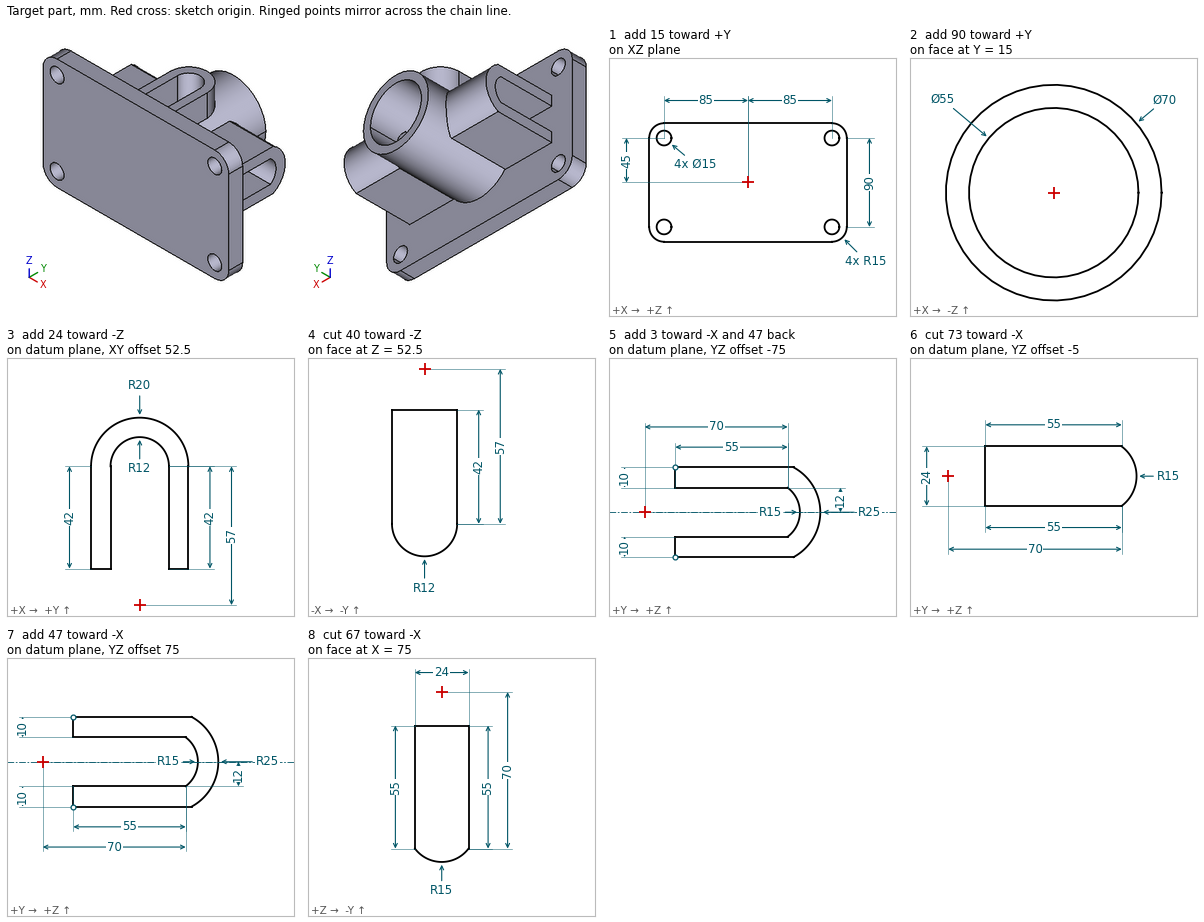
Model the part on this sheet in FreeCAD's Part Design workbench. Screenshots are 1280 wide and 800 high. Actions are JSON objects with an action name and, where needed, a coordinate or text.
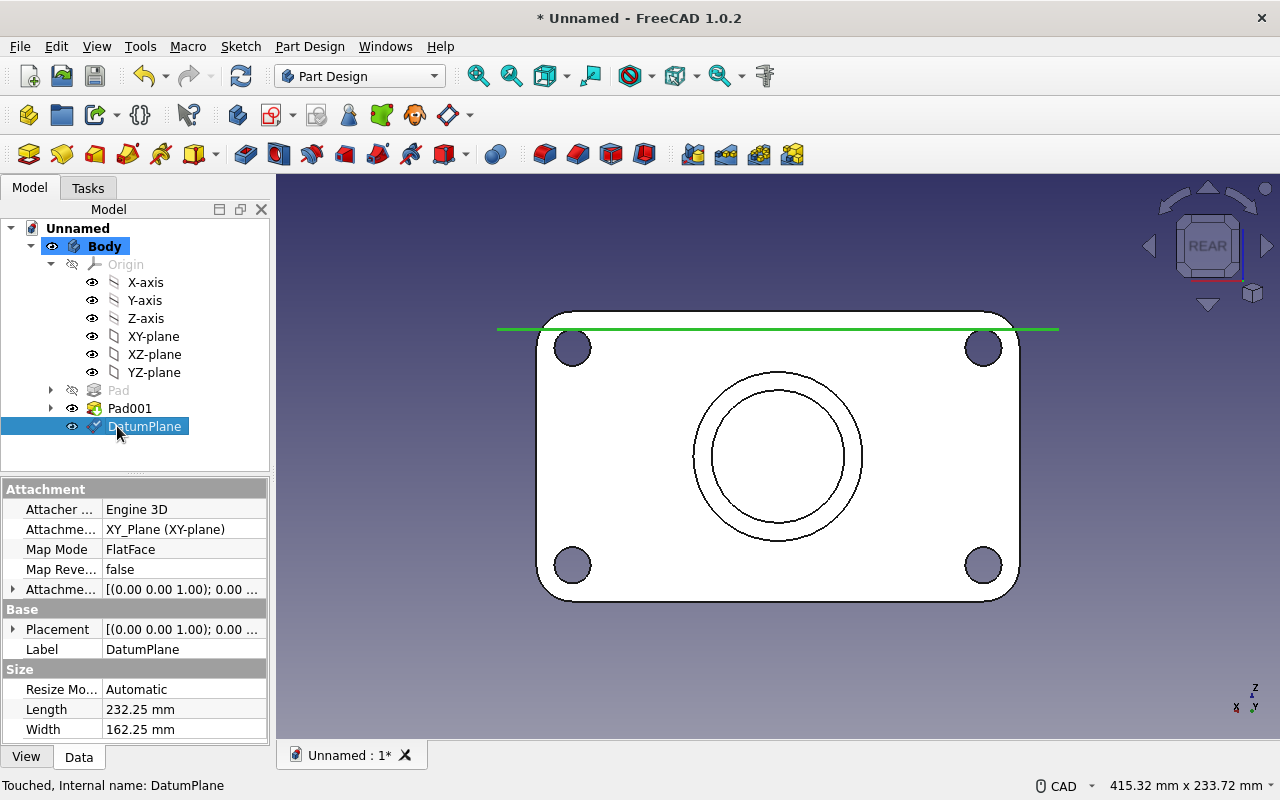
{"action": "left_click", "coordinate": [270, 116]}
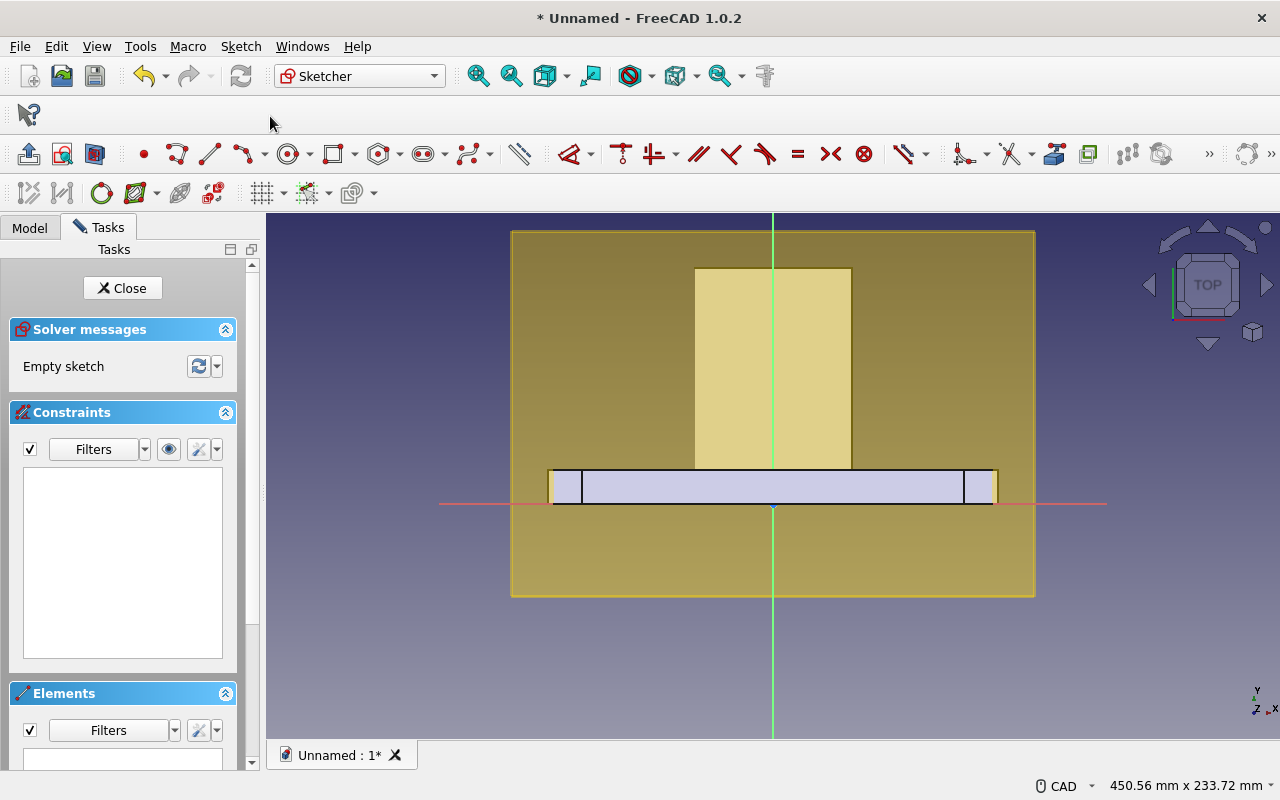
{"action": "key", "text": "q s"}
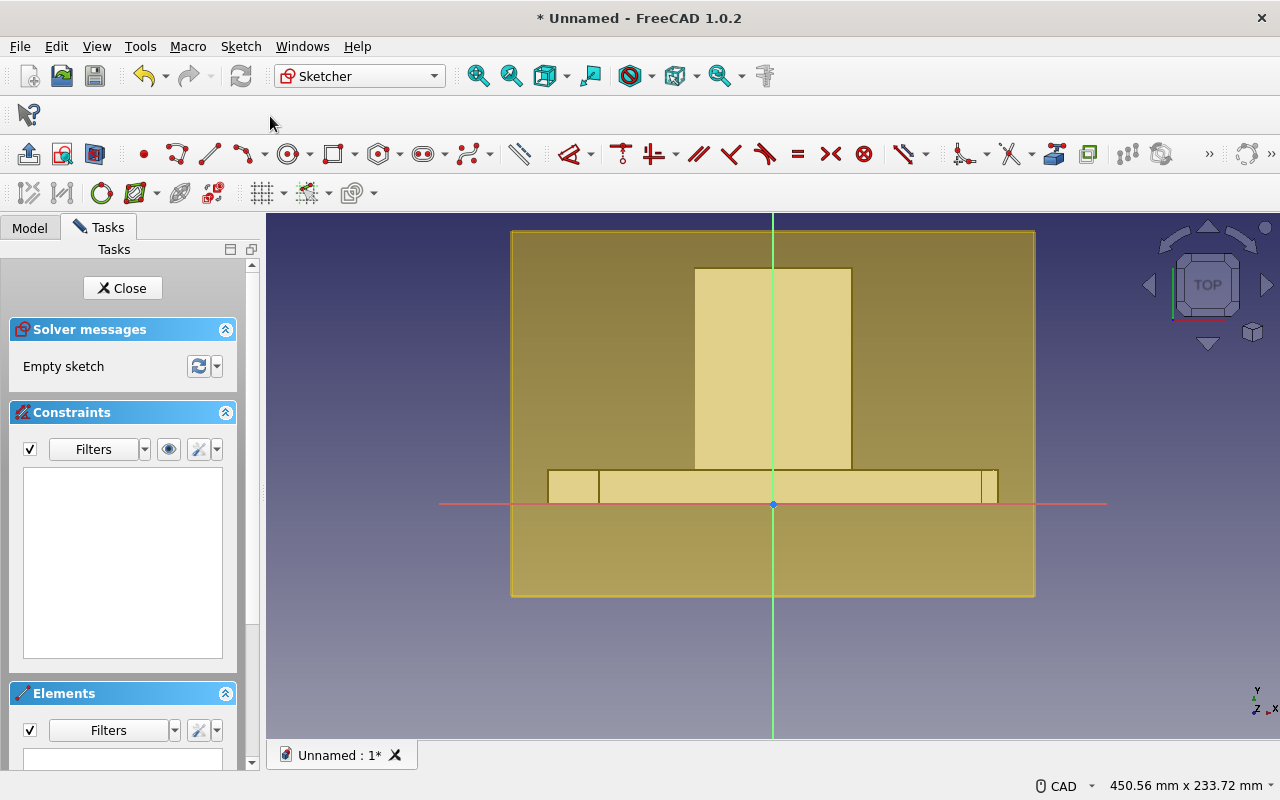
{"action": "scroll", "coordinate": [856, 346], "scroll_direction": "up", "scroll_amount": 3}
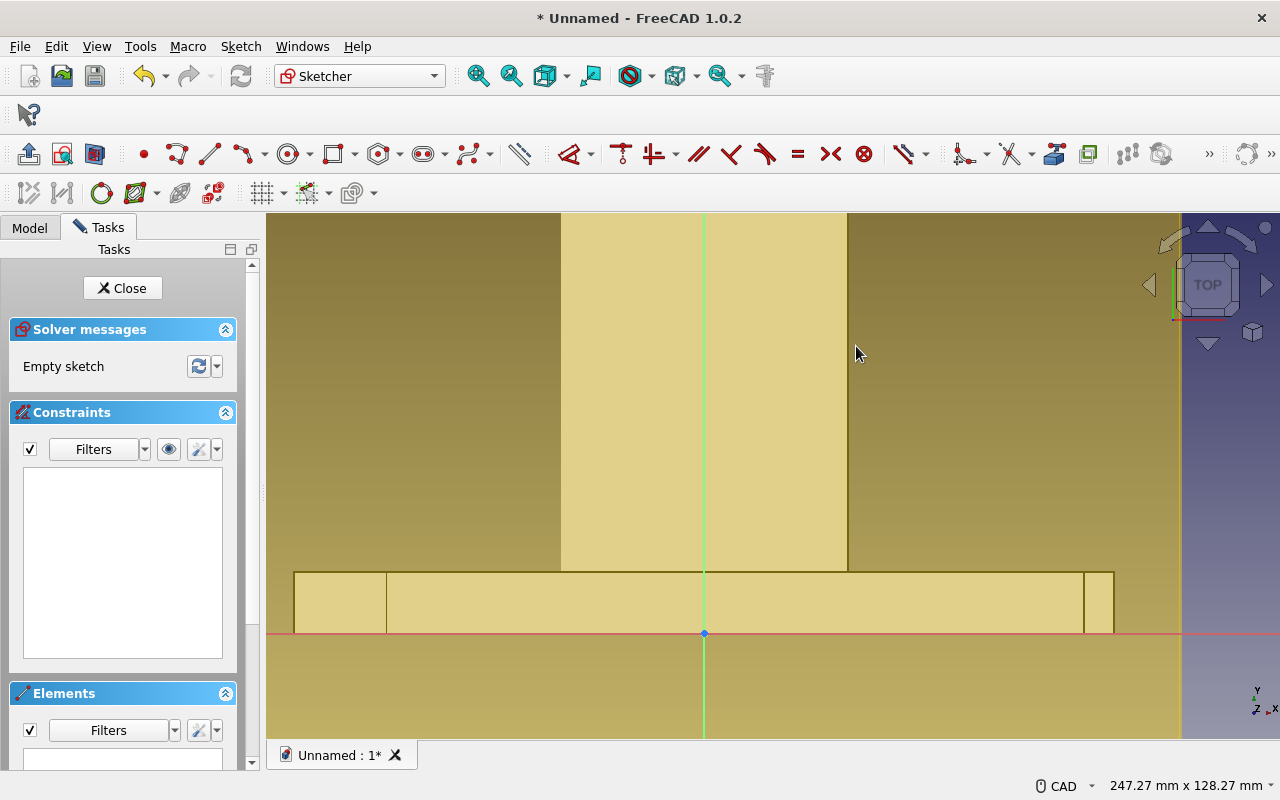
{"action": "key", "text": "g m"}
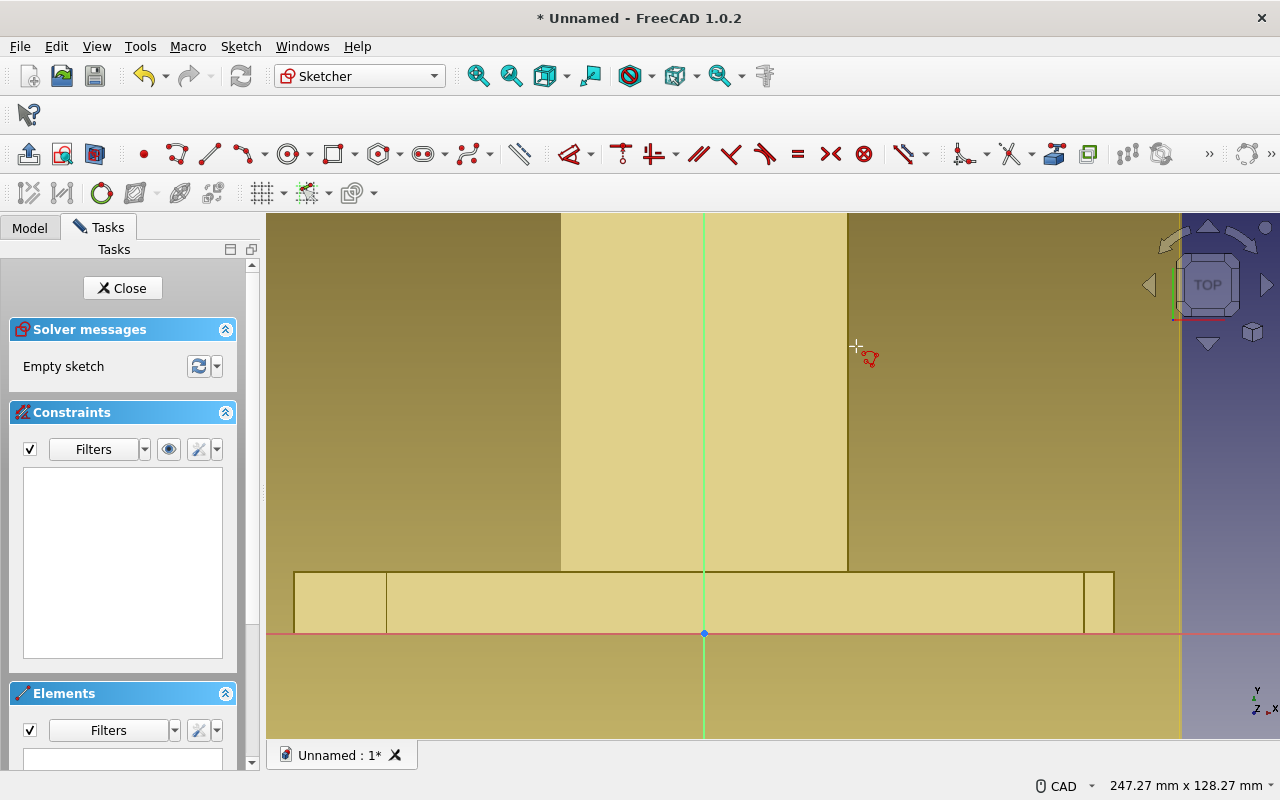
{"action": "left_click", "coordinate": [753, 400]}
{"action": "left_click", "coordinate": [753, 572]}
{"action": "left_click", "coordinate": [786, 572]}
{"action": "left_click", "coordinate": [786, 400]}
{"action": "right_click", "coordinate": [786, 400]}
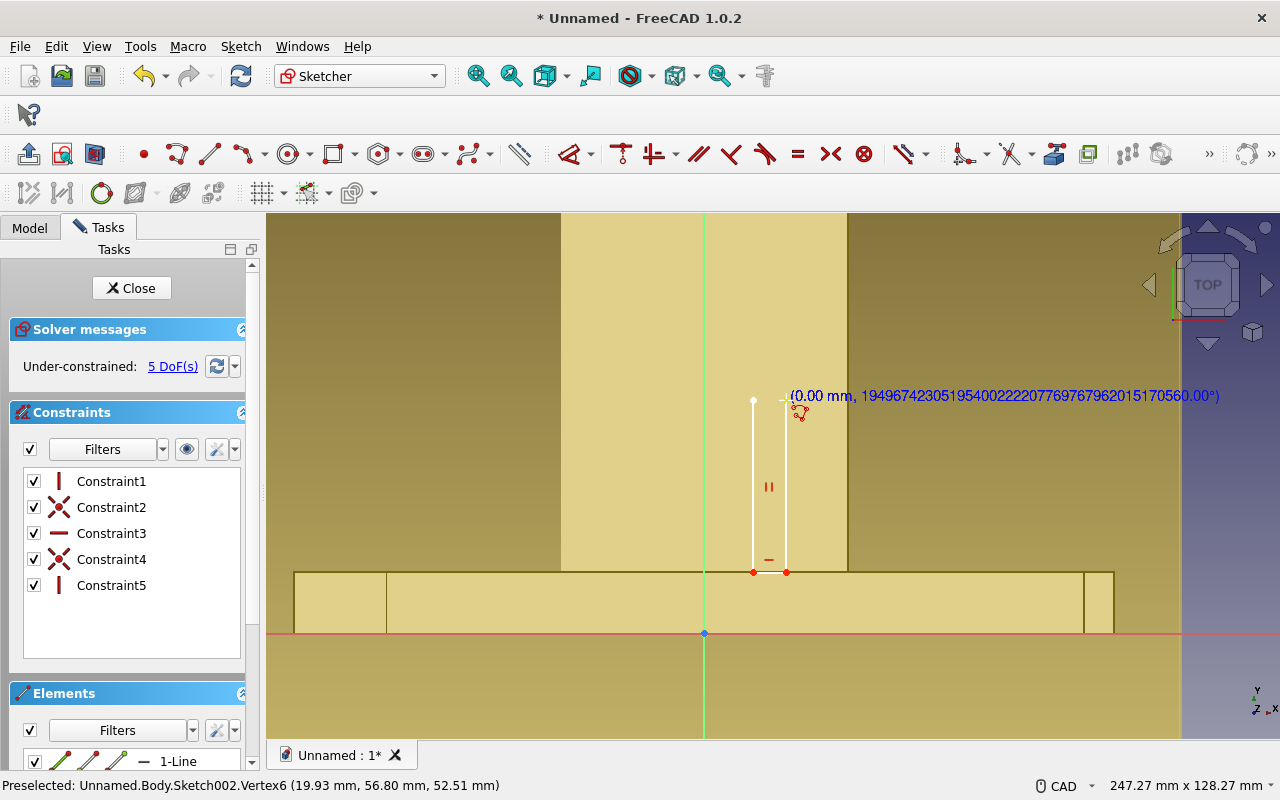
{"action": "left_click", "coordinate": [622, 400]}
{"action": "left_click", "coordinate": [622, 572]}
{"action": "left_click", "coordinate": [655, 572]}
{"action": "left_click", "coordinate": [655, 400]}
{"action": "right_click", "coordinate": [655, 400]}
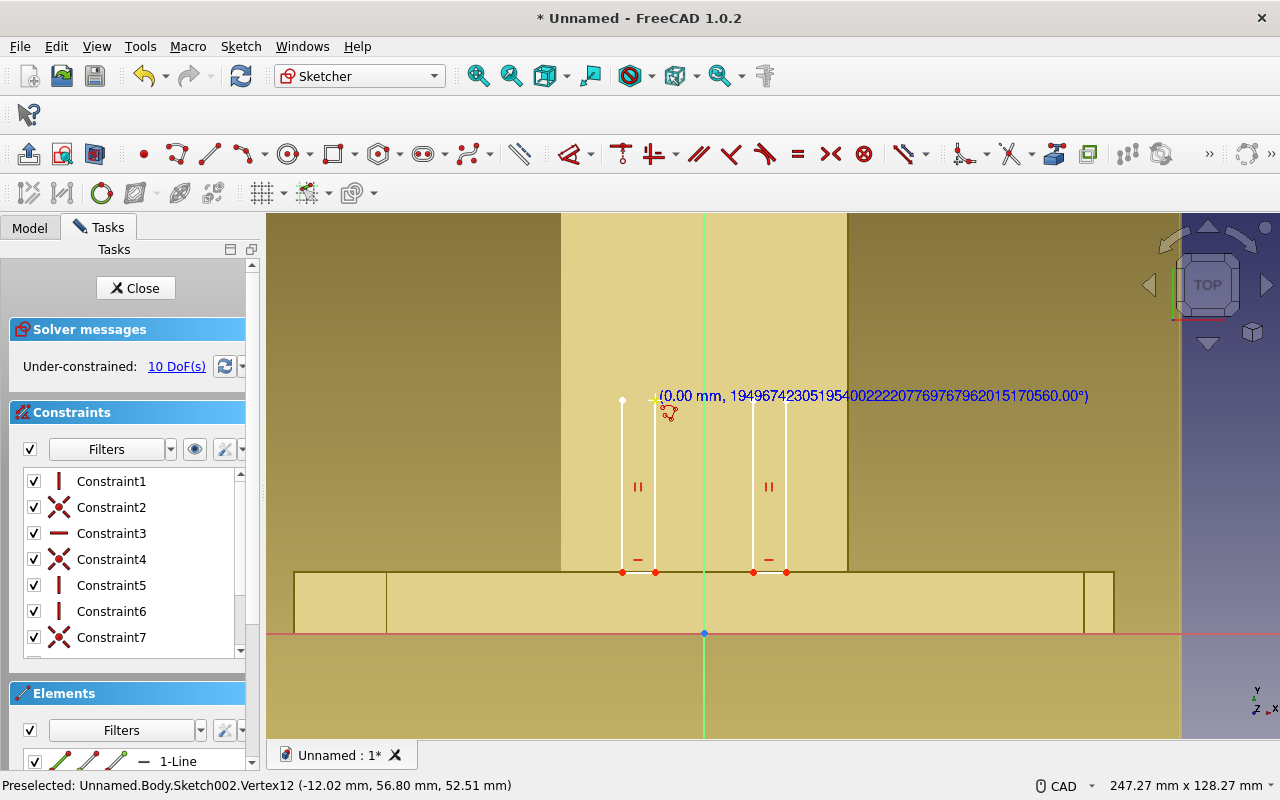
{"action": "left_click", "coordinate": [242, 154]}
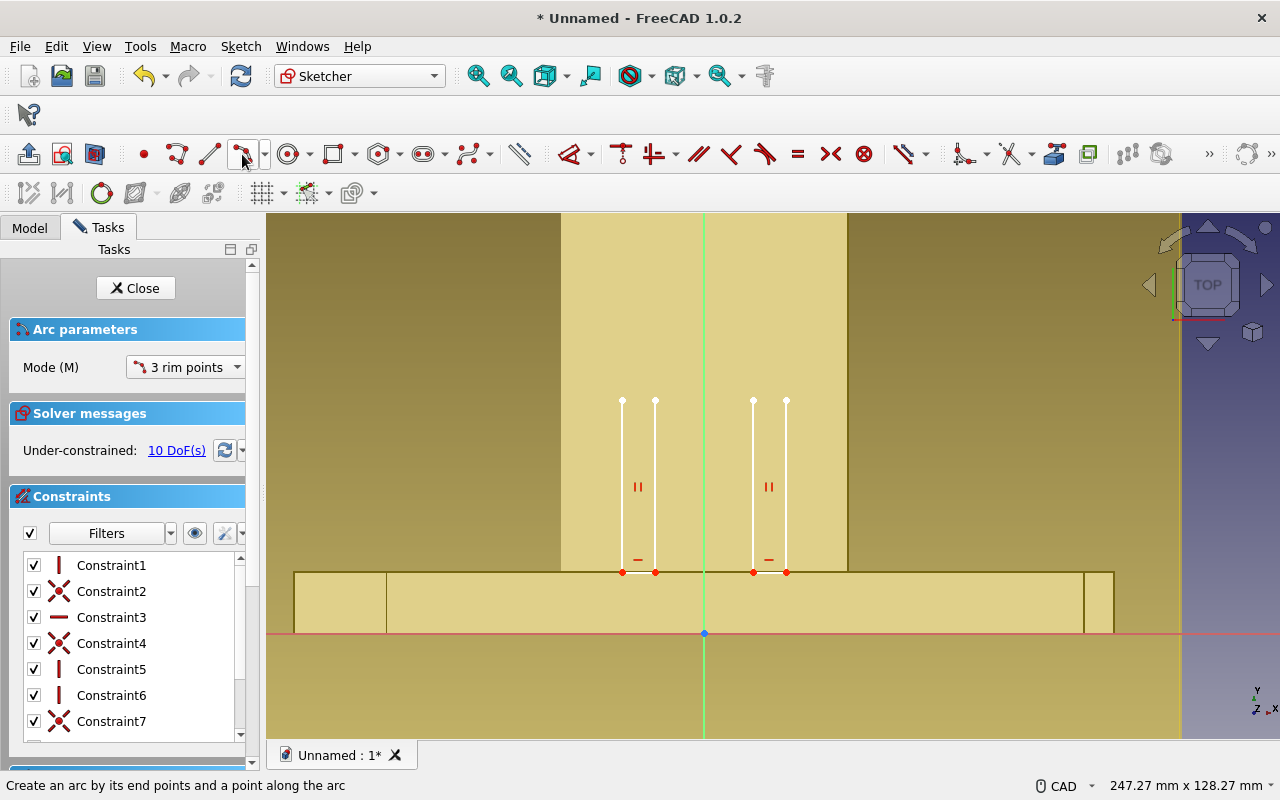
{"action": "left_click", "coordinate": [786, 401]}
{"action": "left_click", "coordinate": [622, 401]}
{"action": "left_click", "coordinate": [730, 322]}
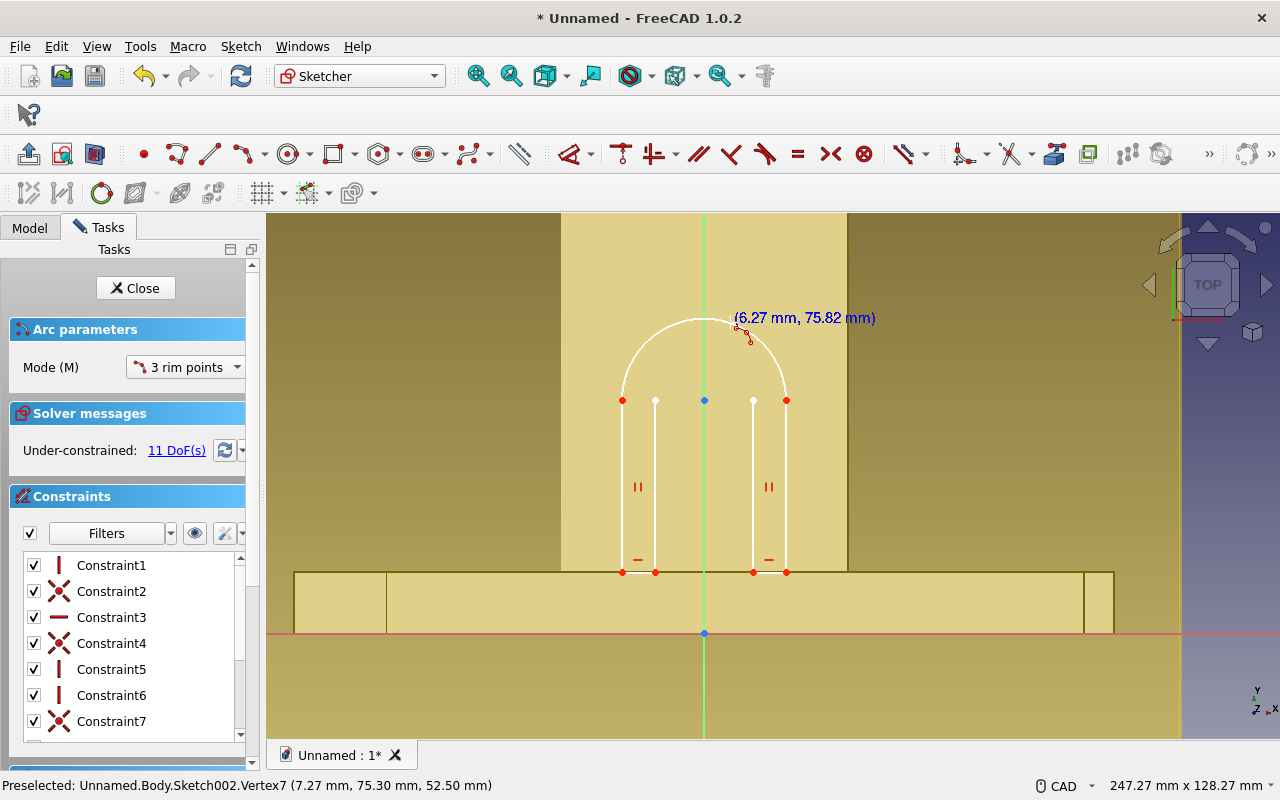
{"action": "left_click", "coordinate": [655, 401]}
{"action": "left_click", "coordinate": [753, 401]}
{"action": "left_click", "coordinate": [719, 353]}
{"action": "key", "text": "Escape"}